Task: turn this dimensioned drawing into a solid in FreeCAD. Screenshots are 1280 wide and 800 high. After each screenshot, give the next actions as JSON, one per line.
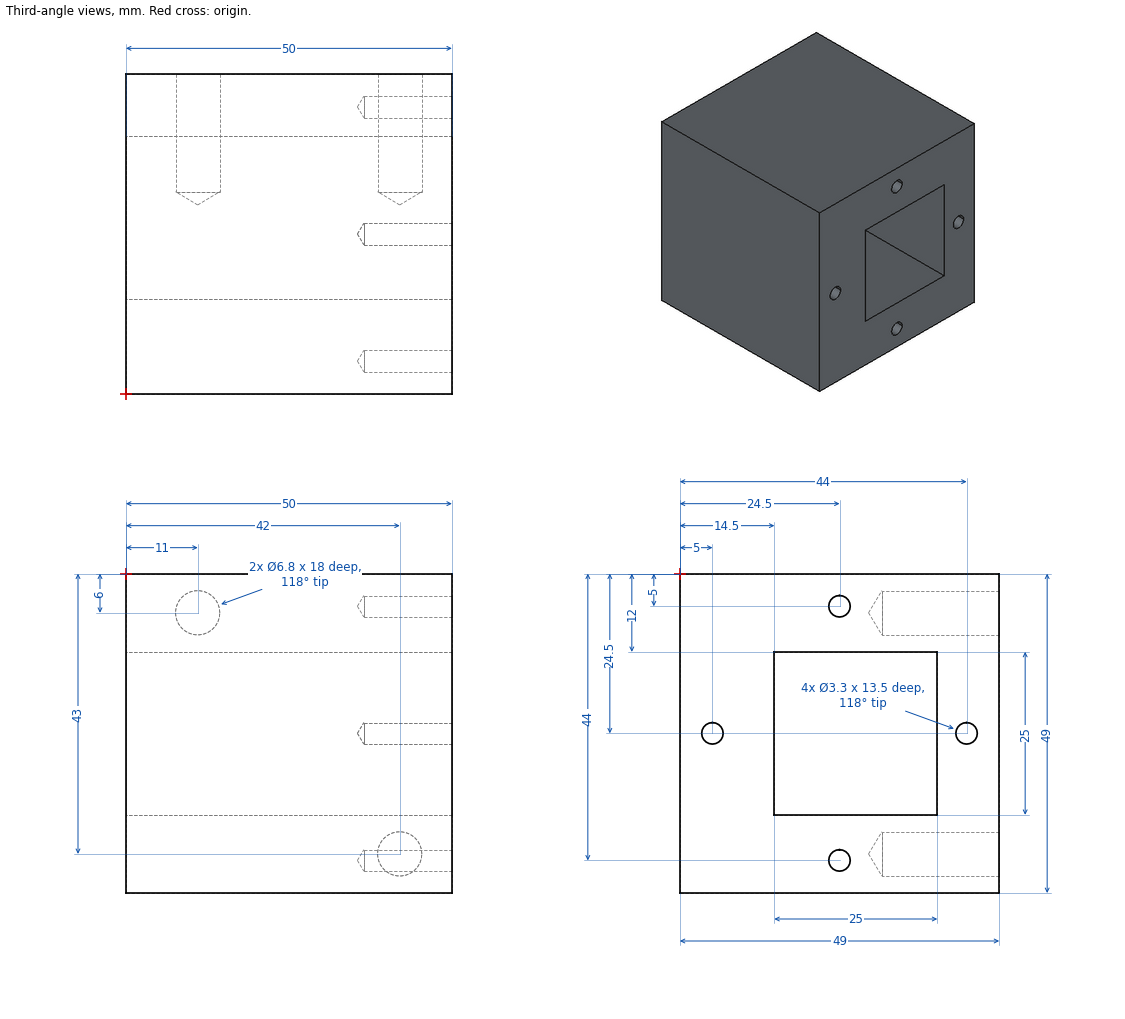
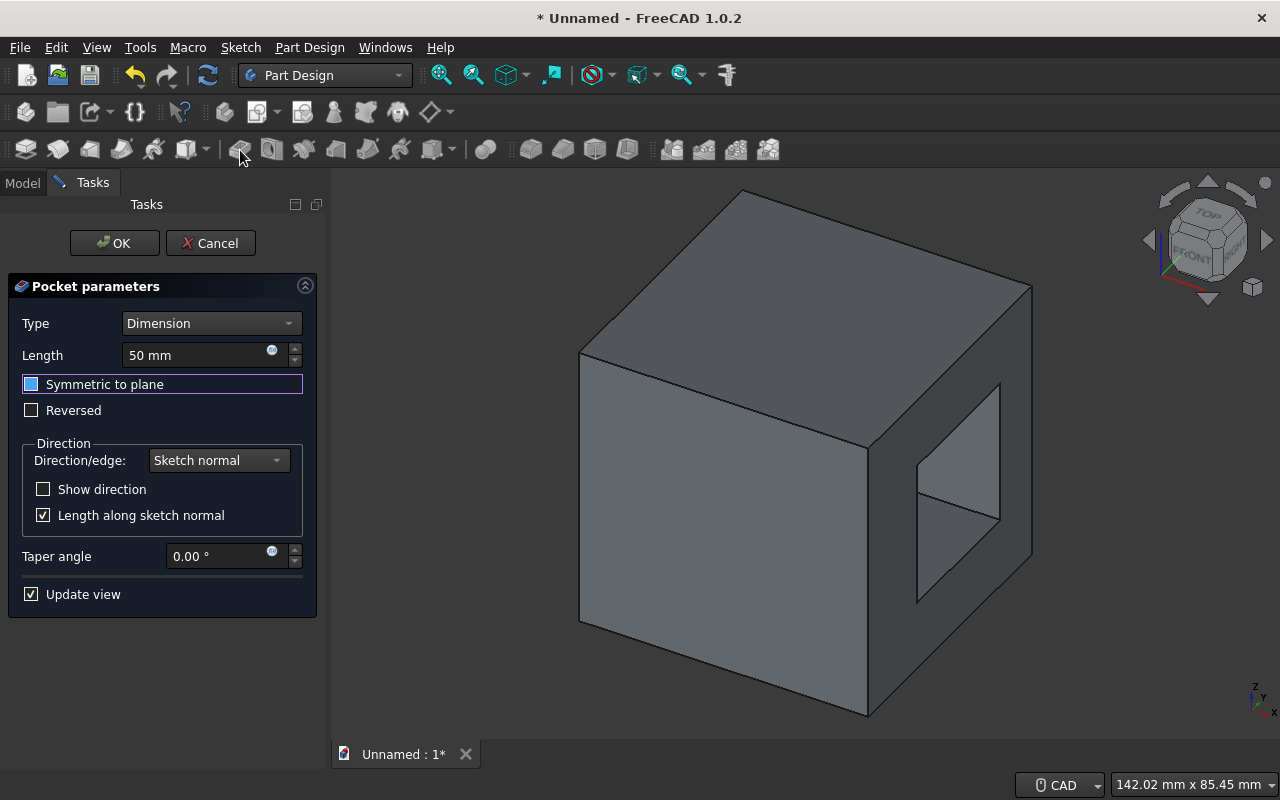
{"action": "left_click", "coordinate": [115, 243]}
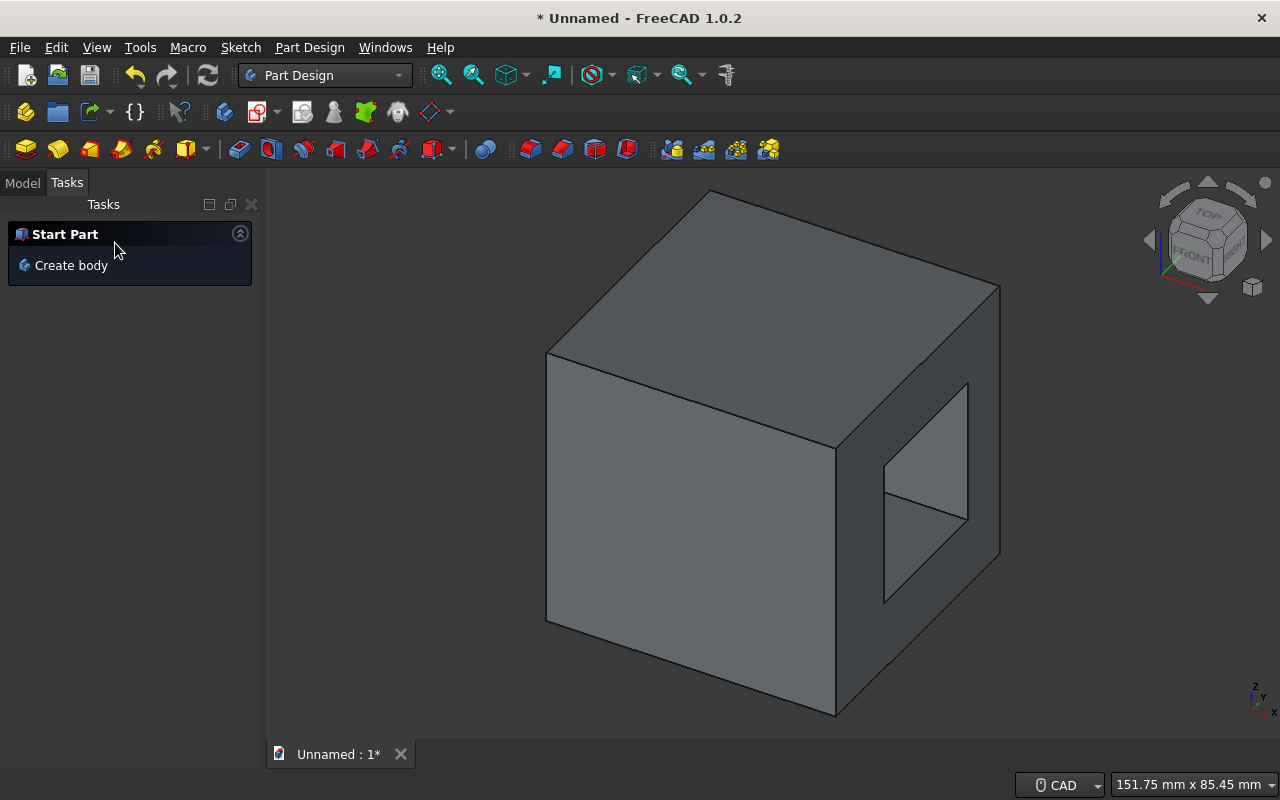
{"action": "left_click", "coordinate": [871, 624]}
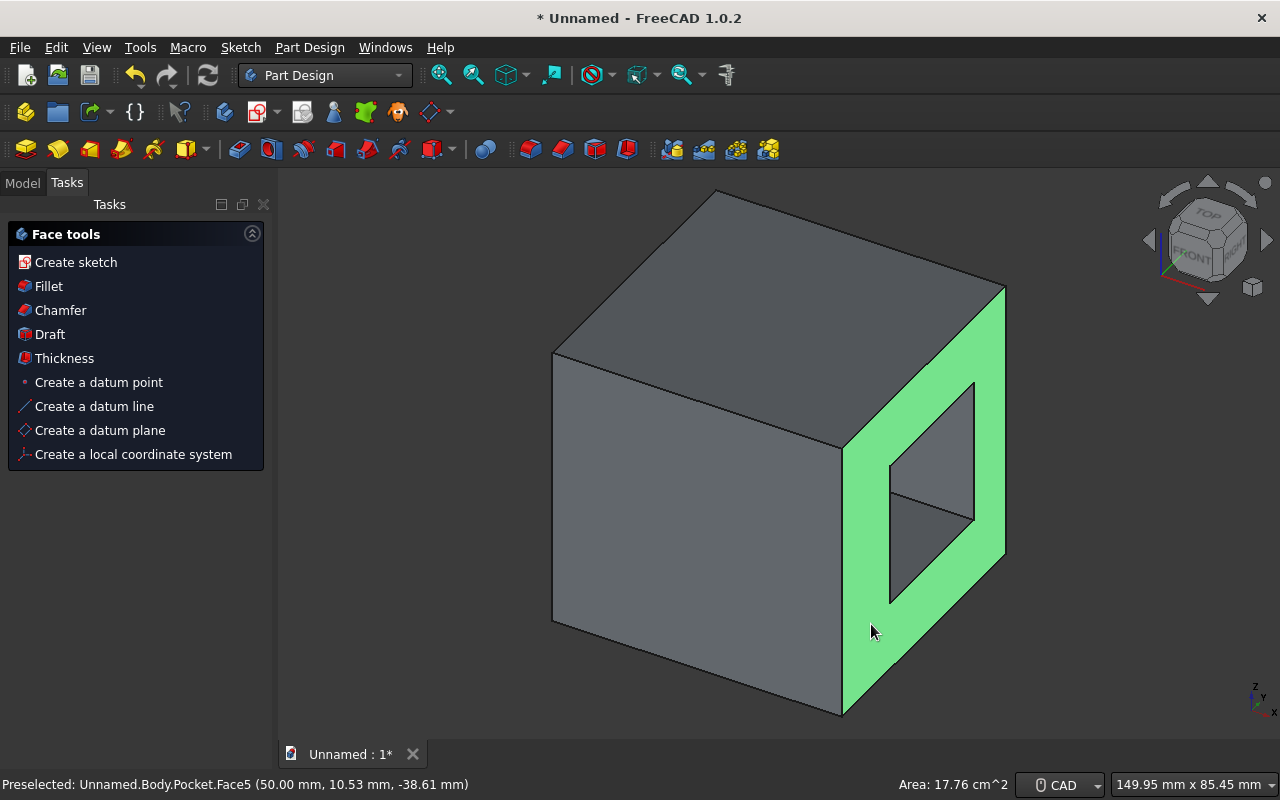
{"action": "left_click", "coordinate": [258, 112]}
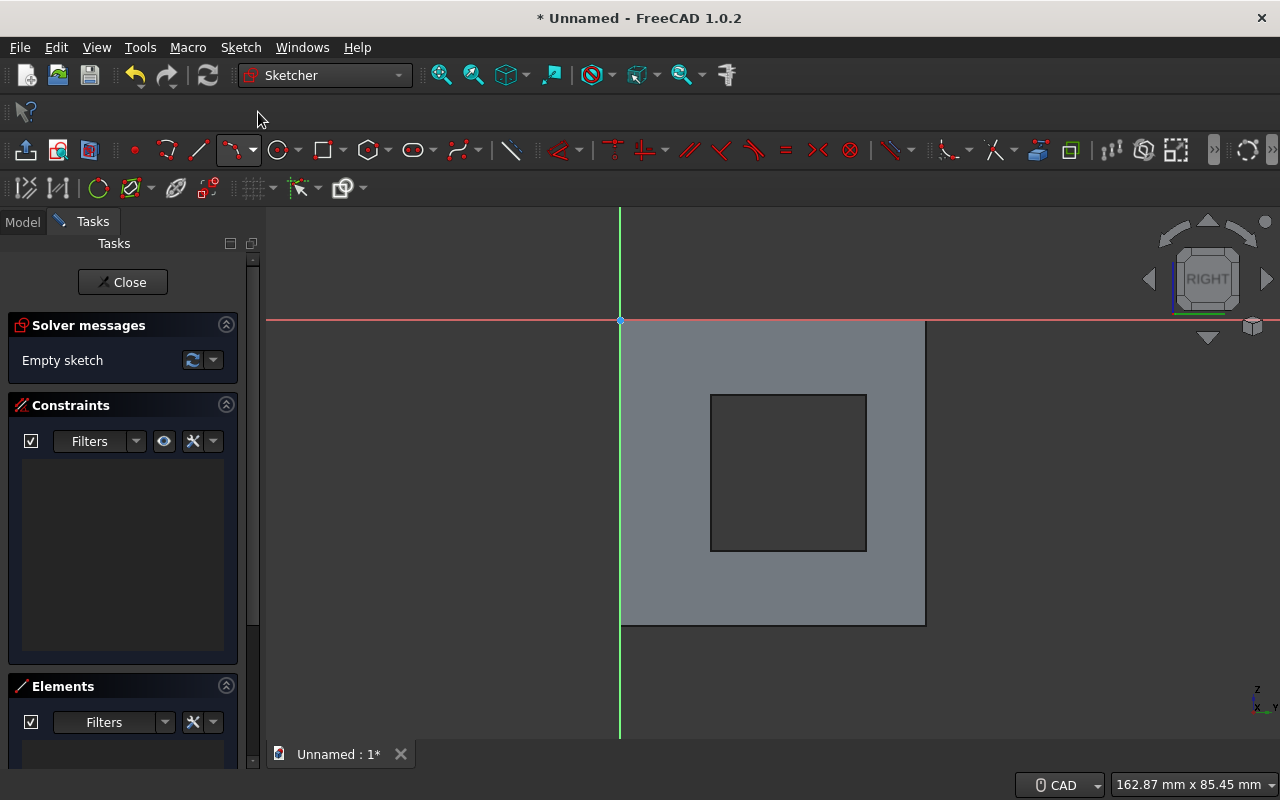
{"action": "key", "text": "g c"}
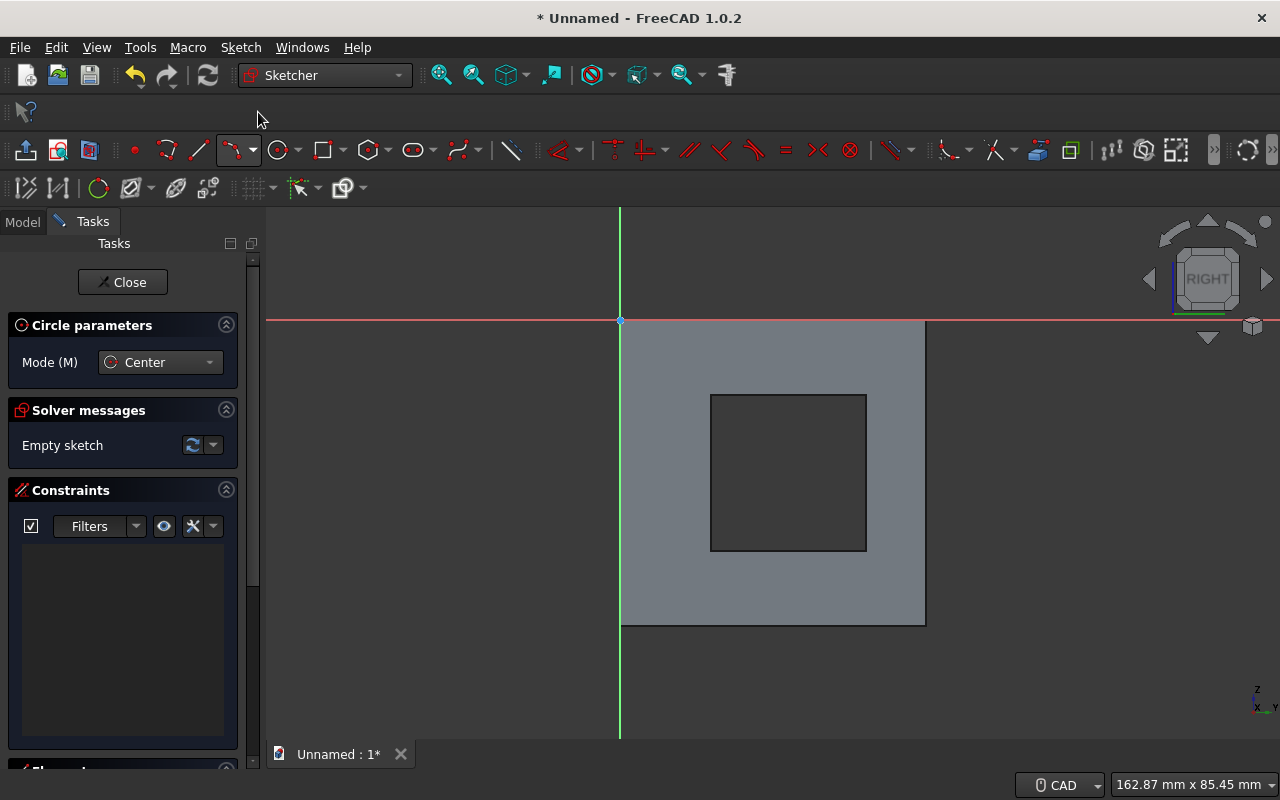
{"action": "scroll", "coordinate": [894, 473], "scroll_direction": "up", "scroll_amount": 4}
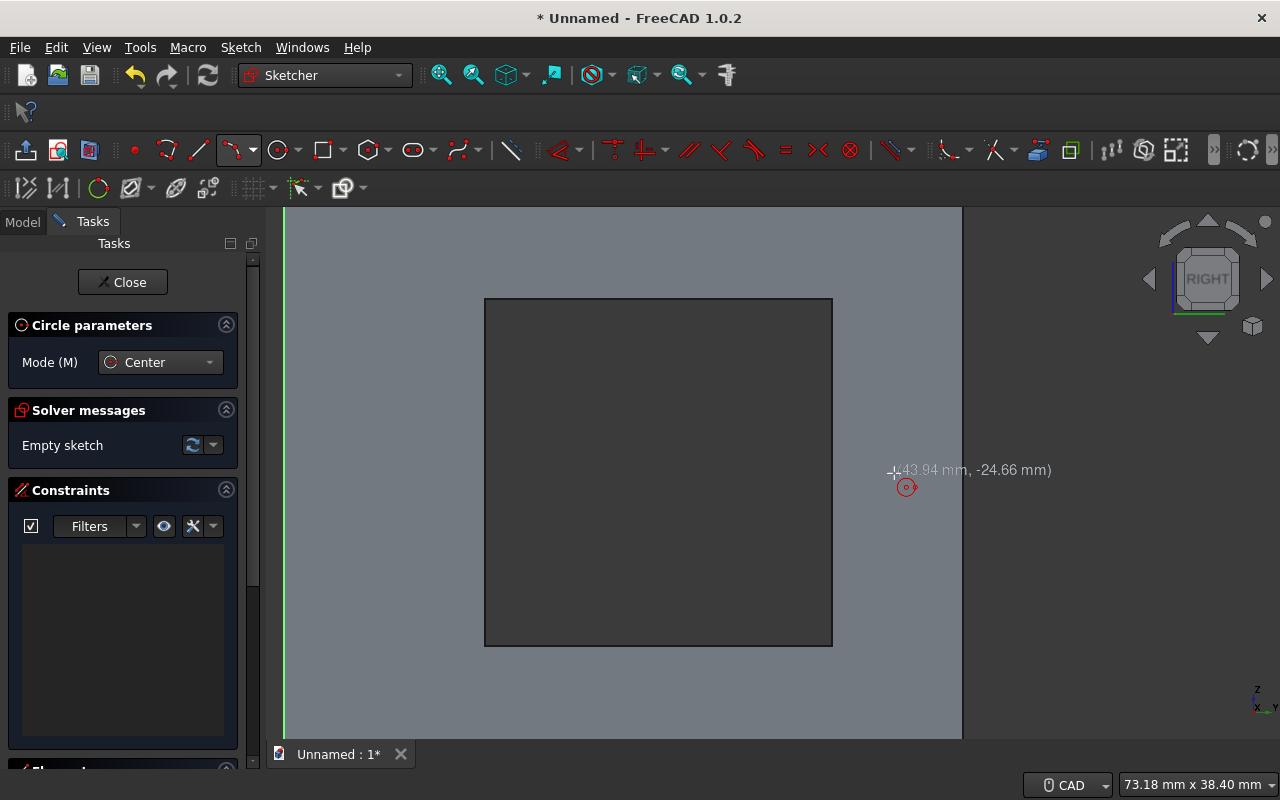
{"action": "left_click", "coordinate": [894, 472]}
{"action": "mouse_move", "coordinate": [910, 456]}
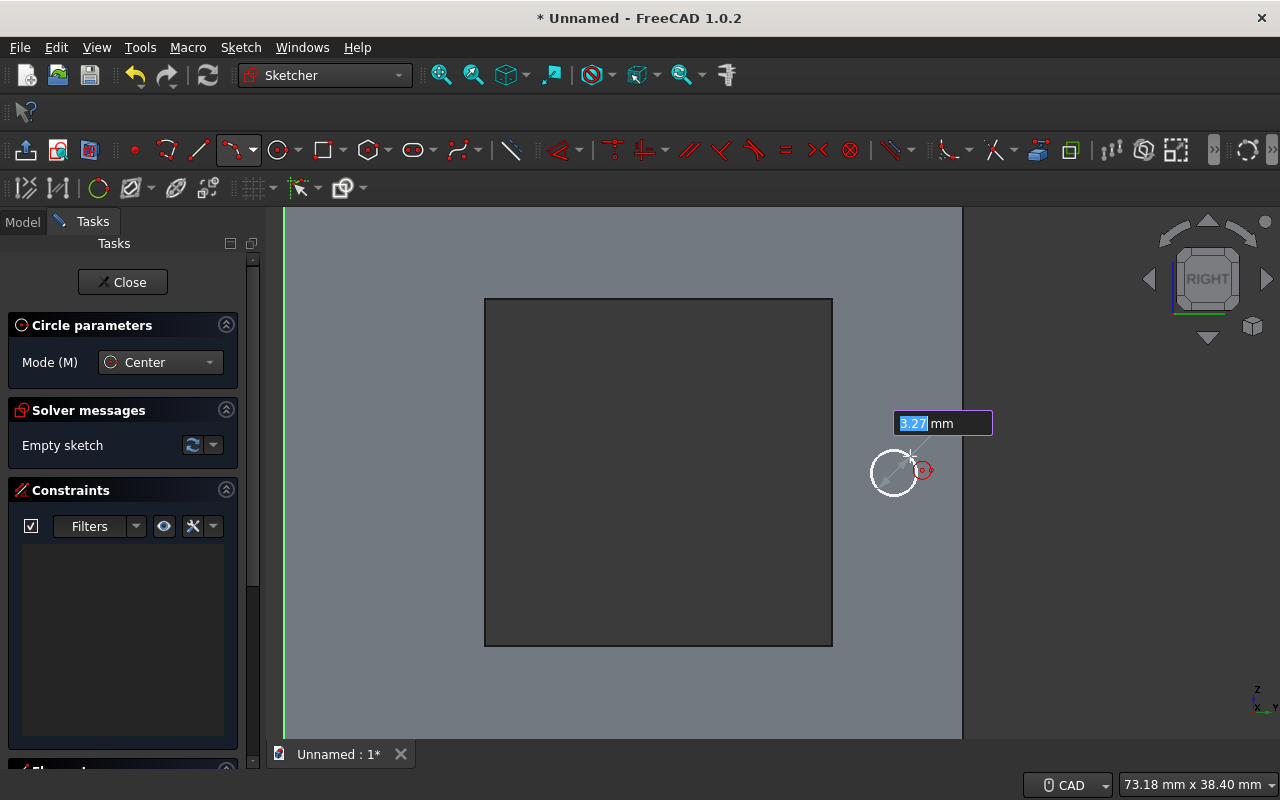
{"action": "type", "text": "3.3"}
{"action": "key", "text": "Return"}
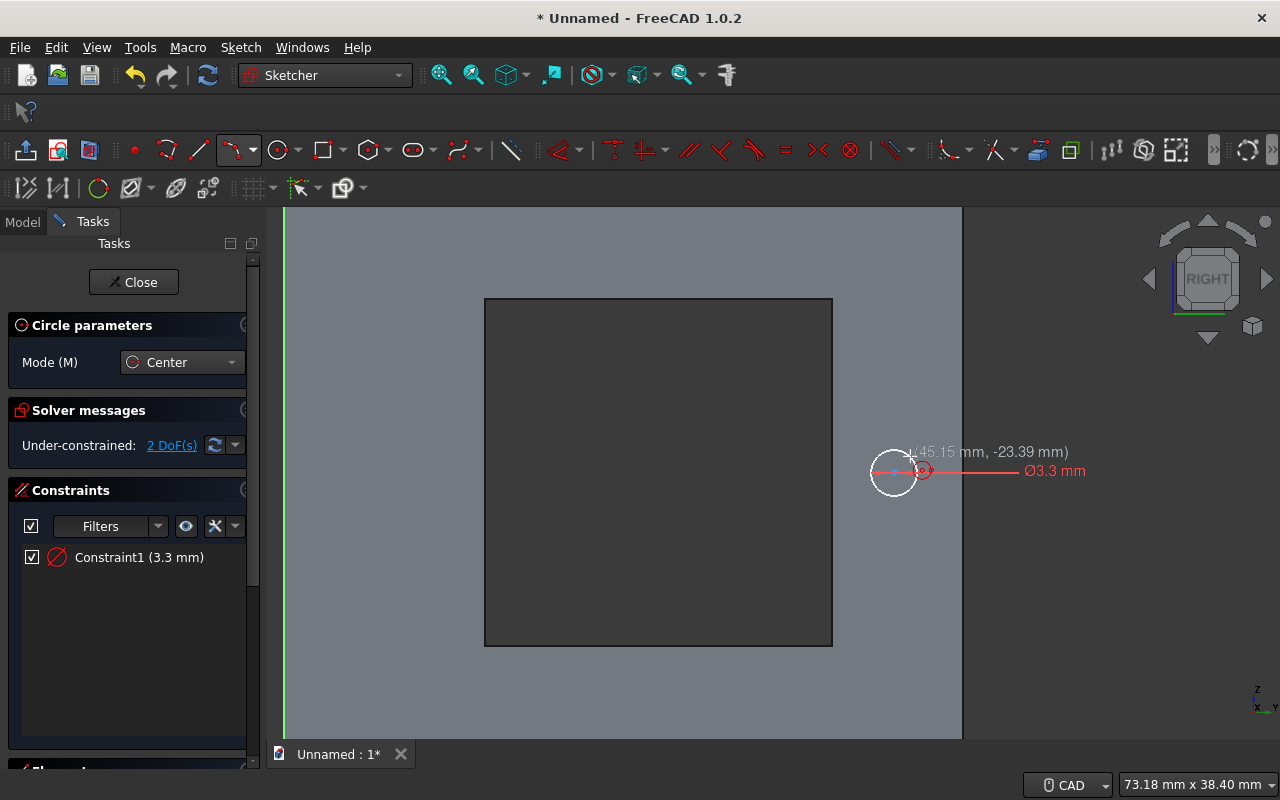
{"action": "scroll", "coordinate": [831, 502], "scroll_direction": "down", "scroll_amount": 3}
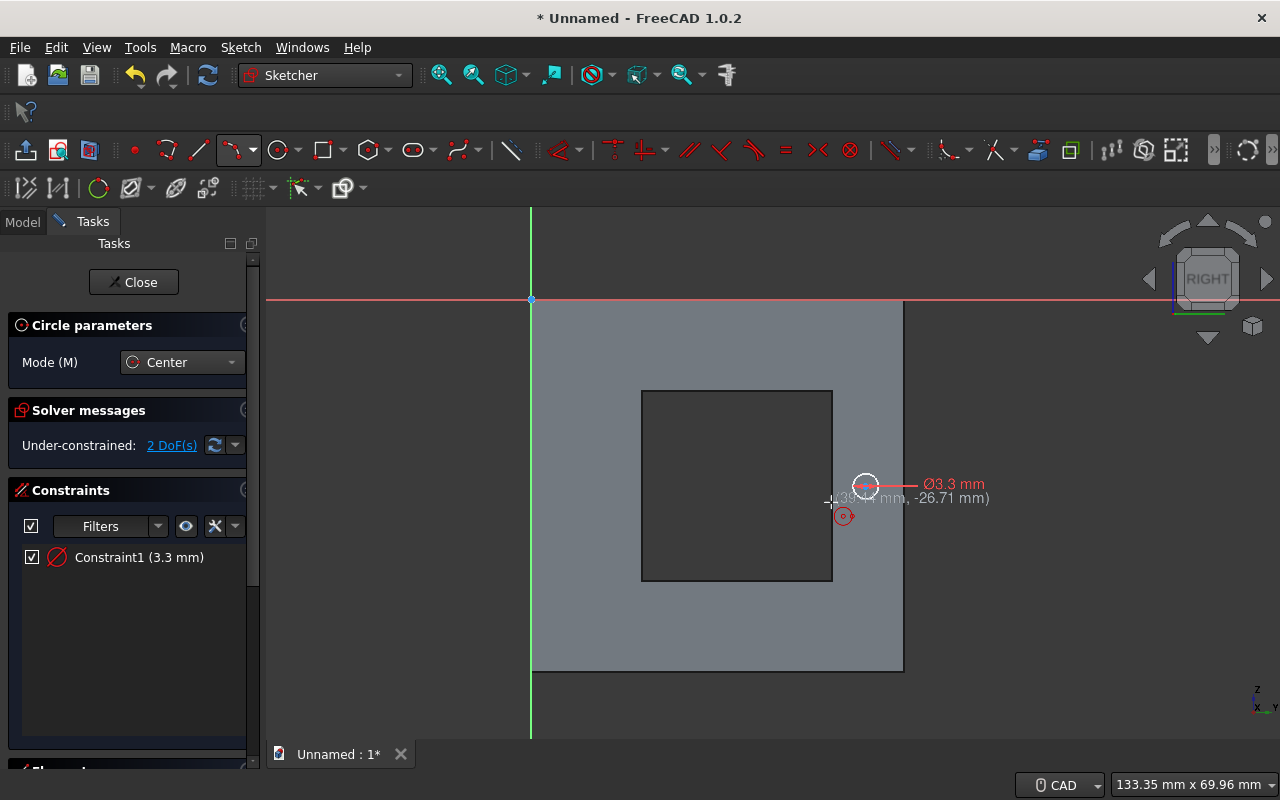
{"action": "scroll", "coordinate": [718, 338], "scroll_direction": "up", "scroll_amount": 3}